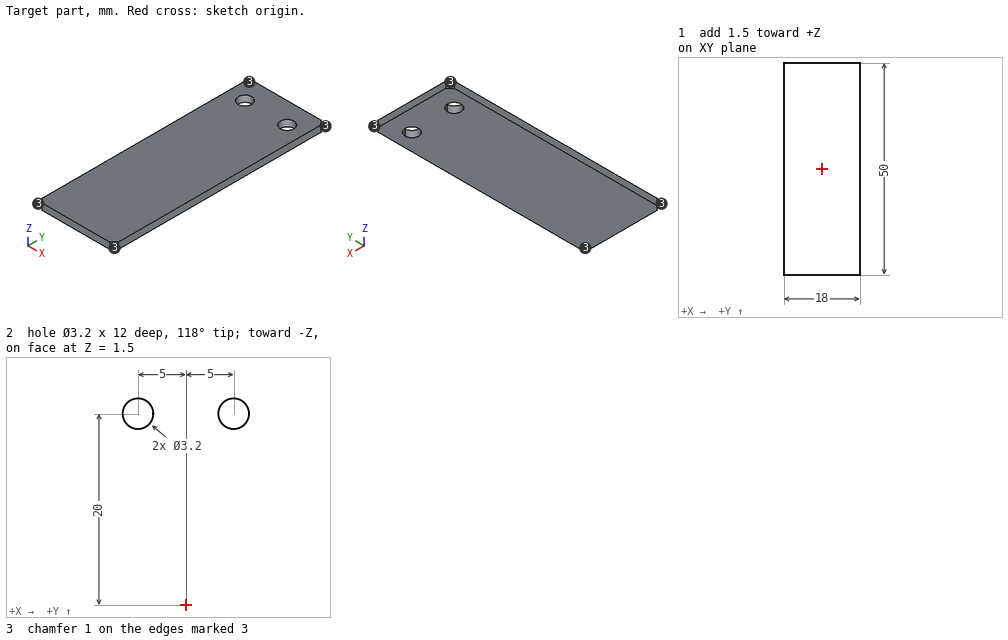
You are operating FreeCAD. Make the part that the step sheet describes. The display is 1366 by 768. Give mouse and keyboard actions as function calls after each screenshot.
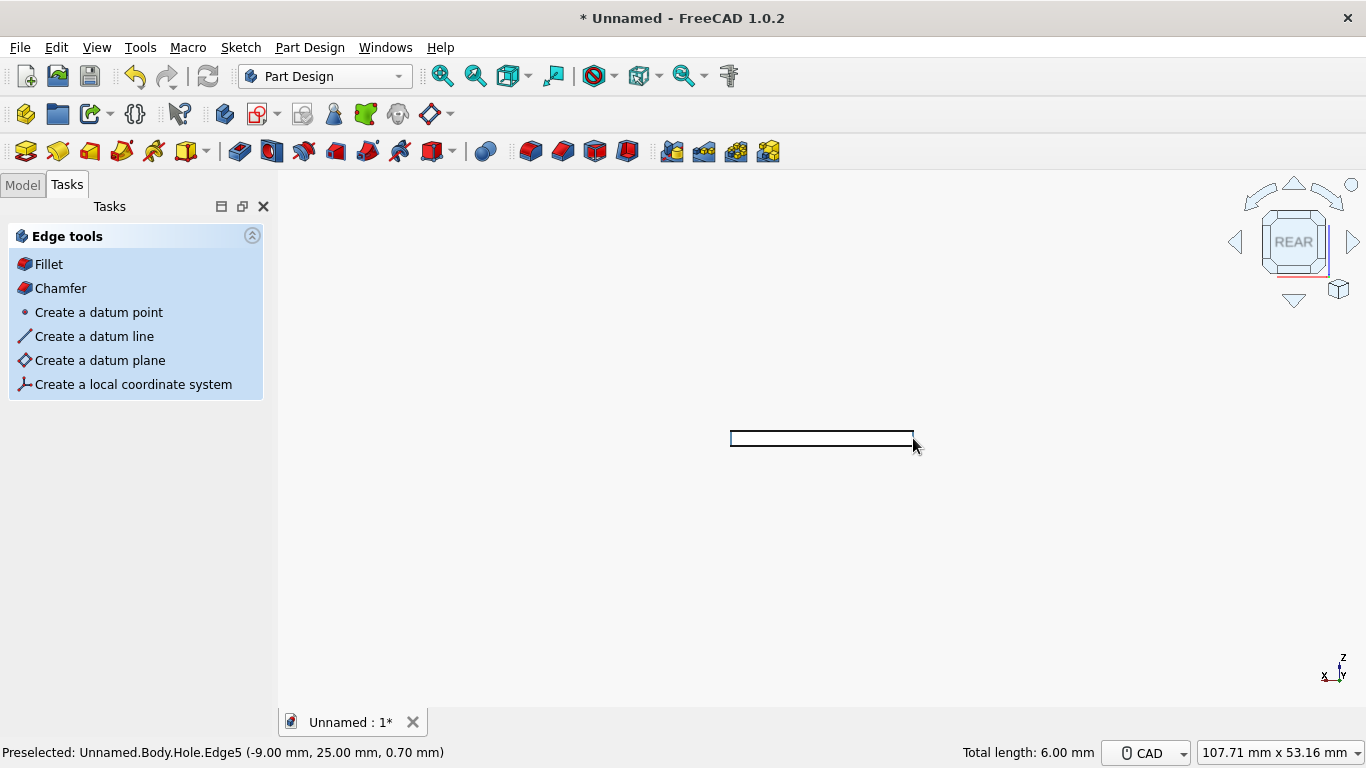
click(564, 152)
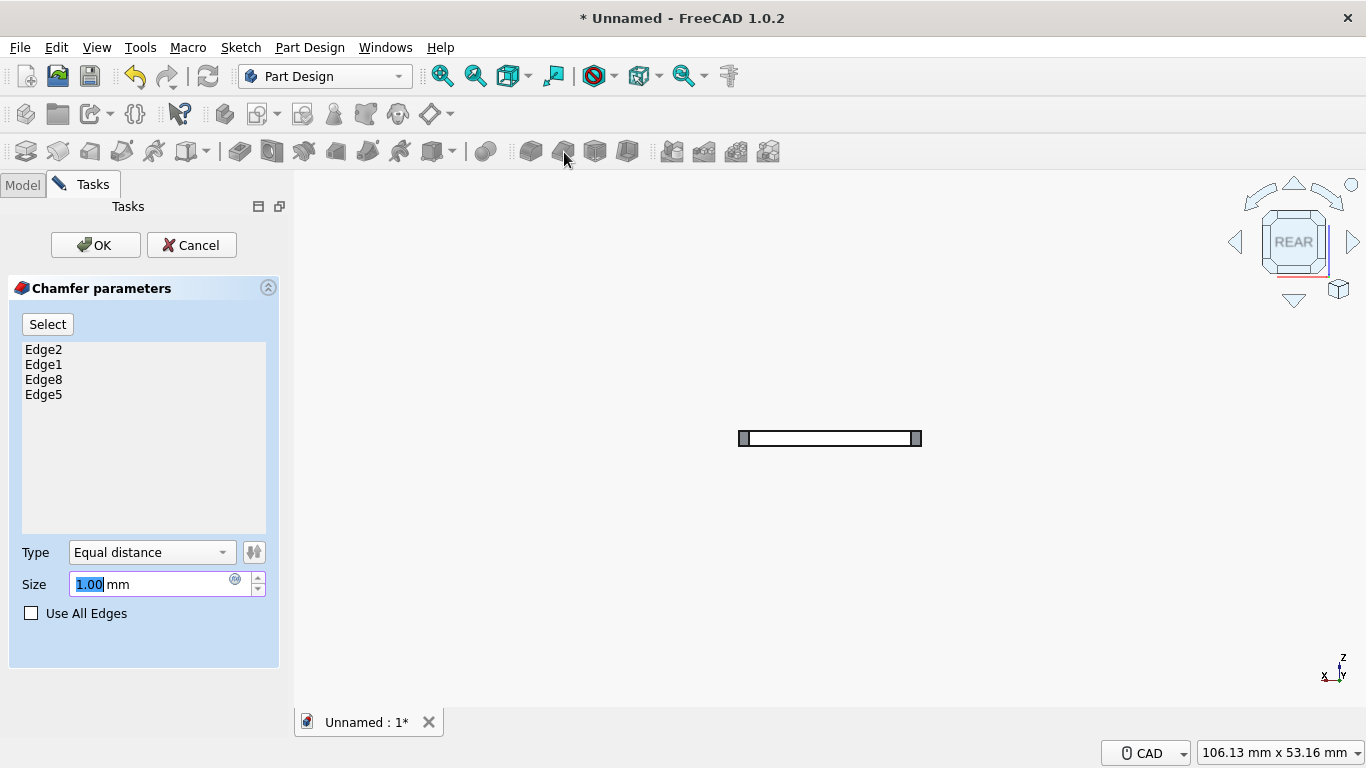
text(1)
key(Tab)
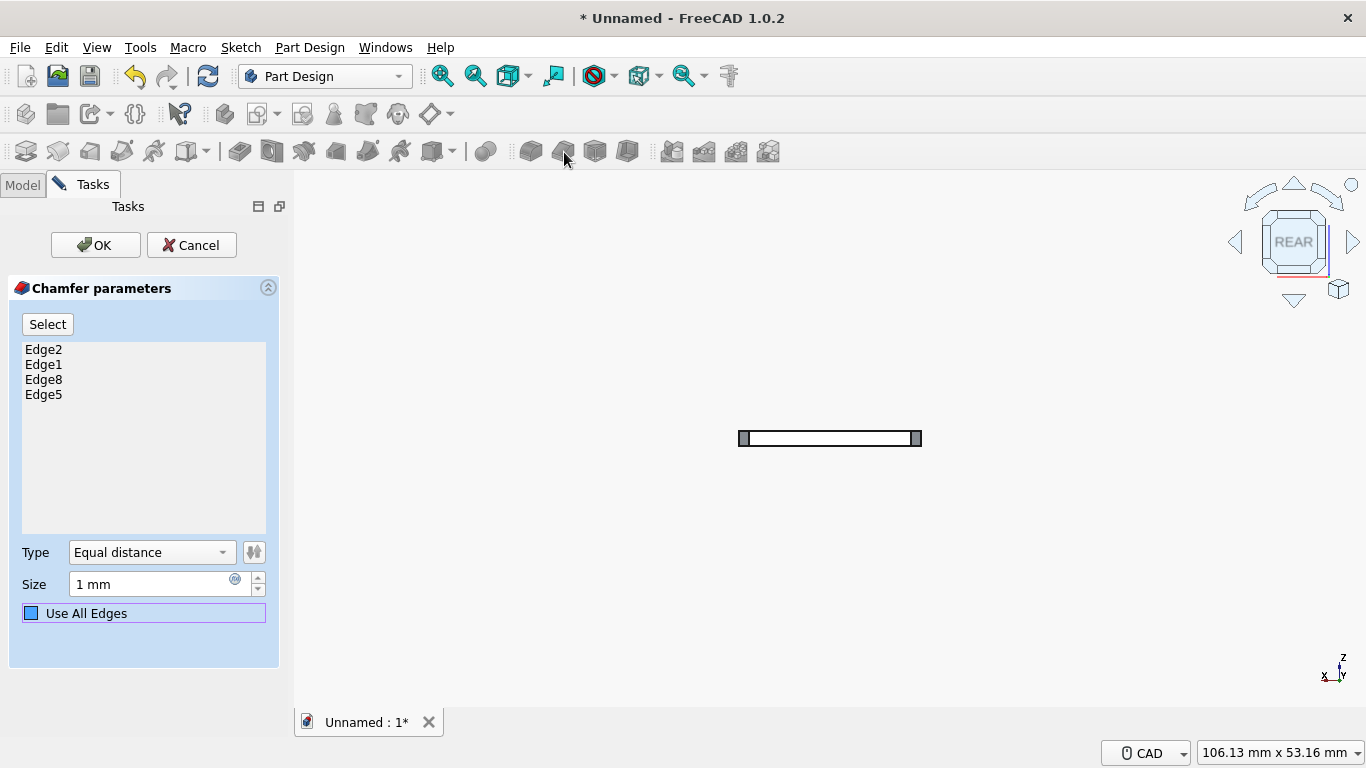
click(96, 245)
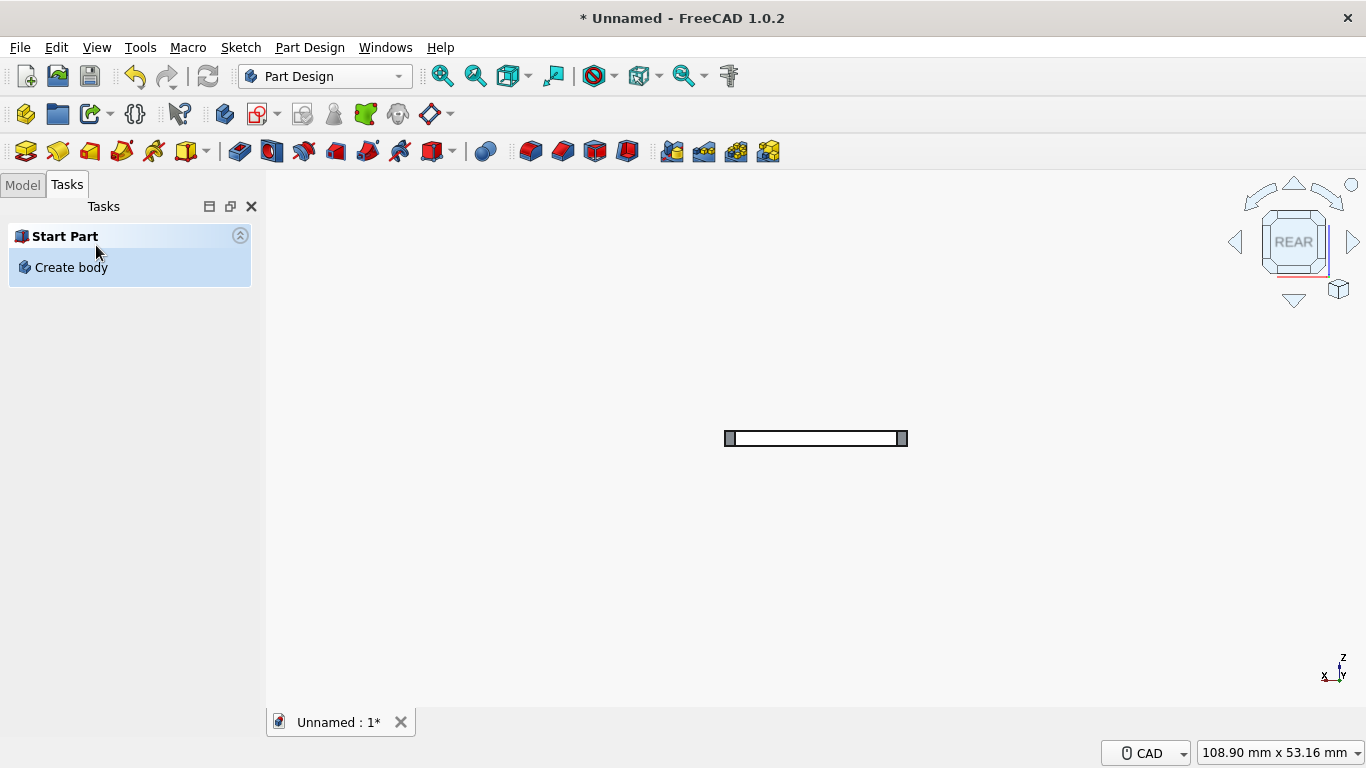
key(0)